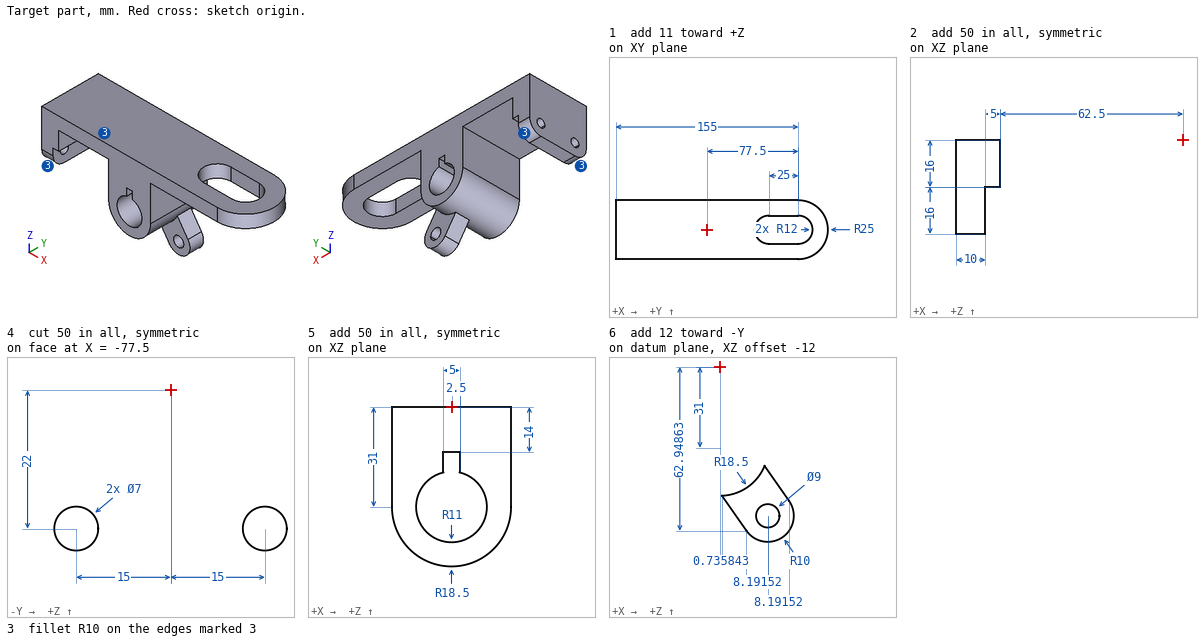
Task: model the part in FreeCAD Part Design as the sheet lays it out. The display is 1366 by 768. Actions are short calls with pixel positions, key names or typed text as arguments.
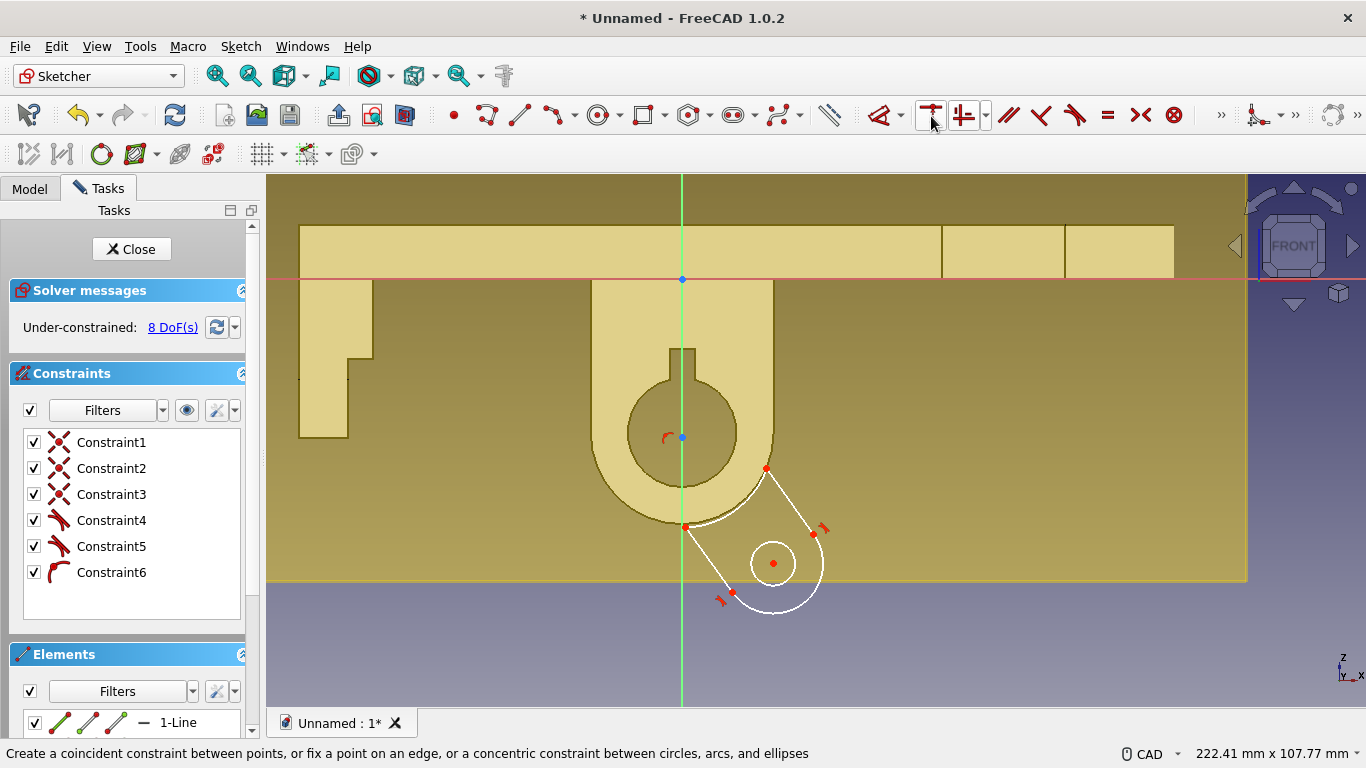
click(878, 116)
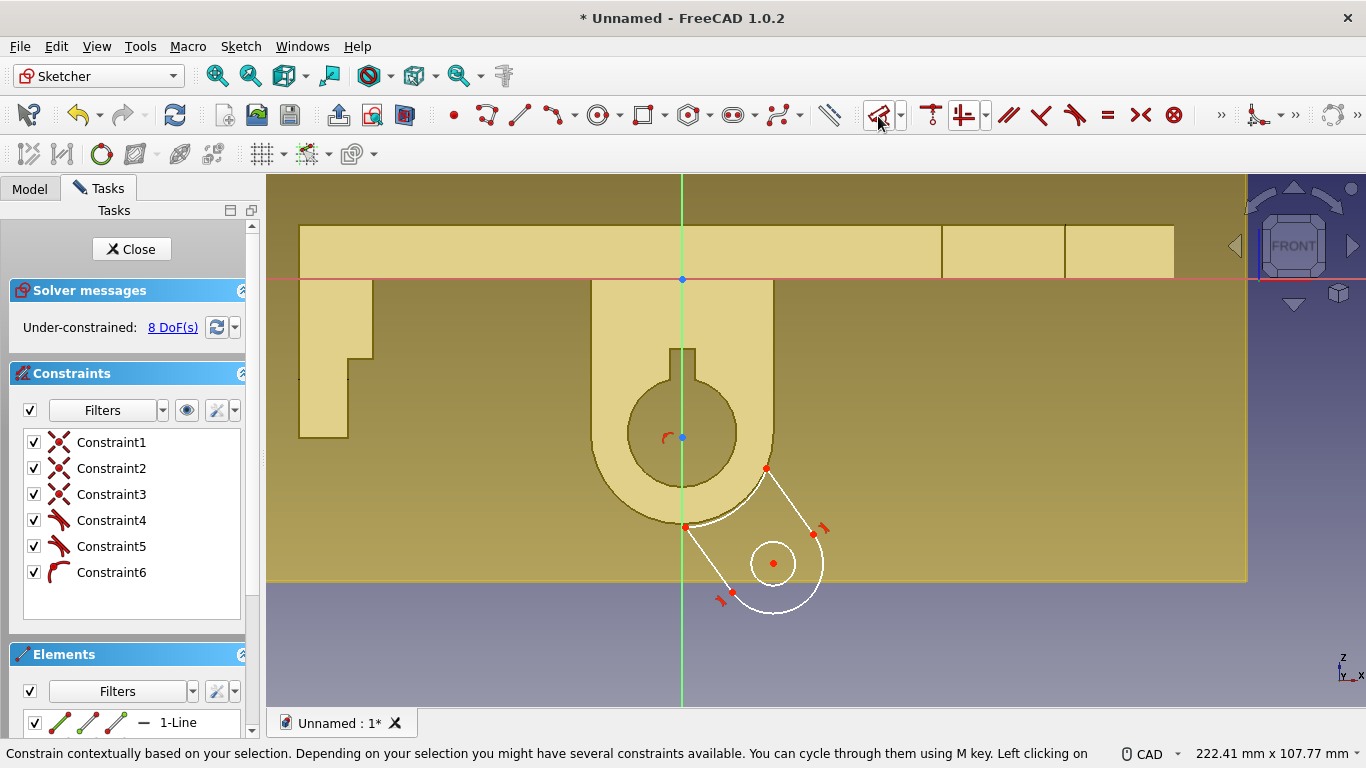
click(773, 614)
click(773, 646)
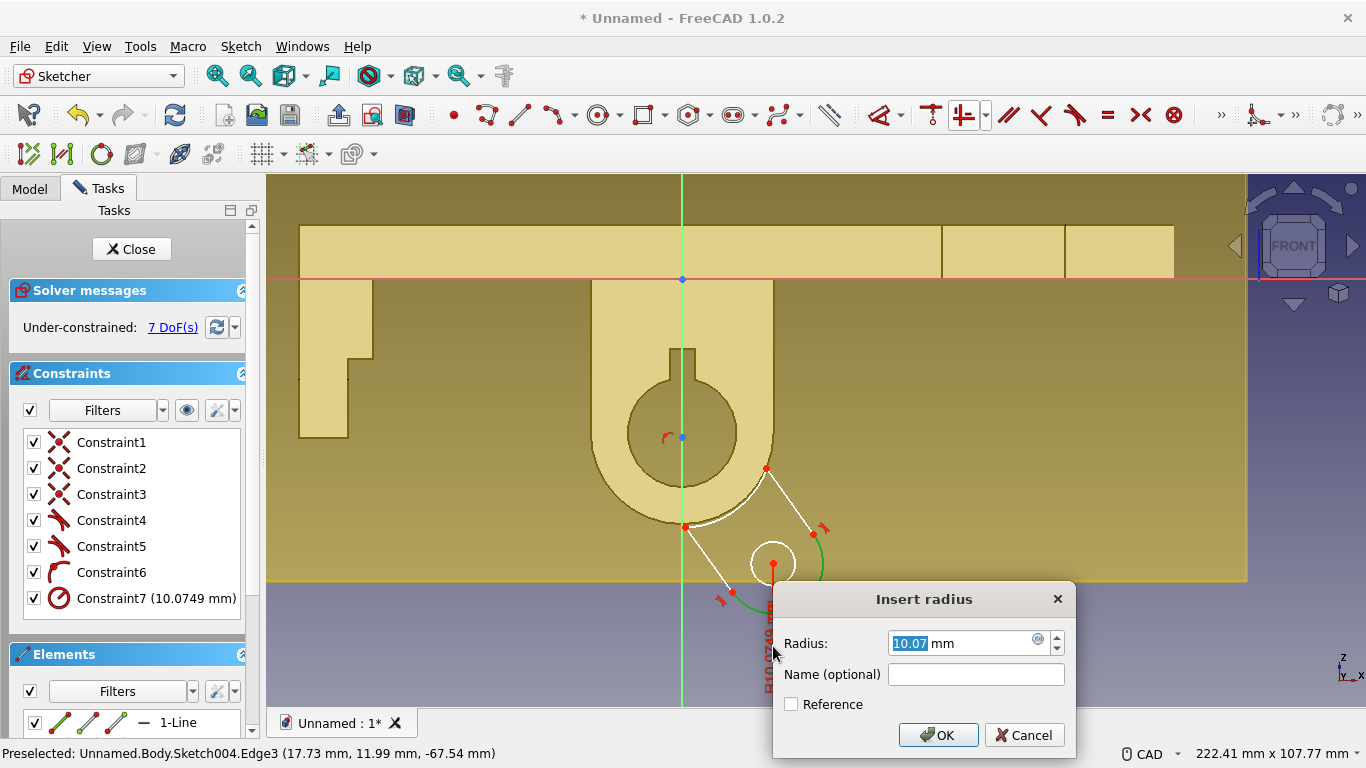
text(10)
key(Return)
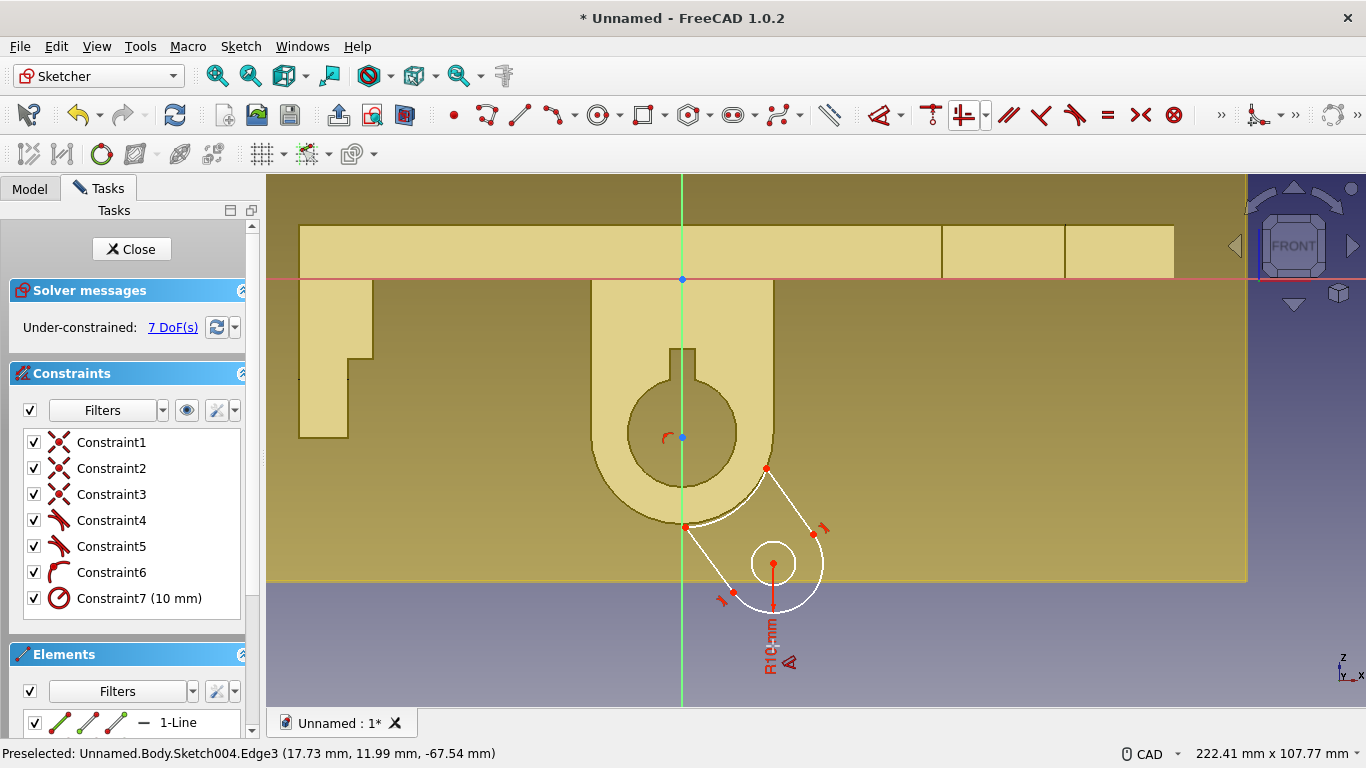
click(717, 521)
click(729, 551)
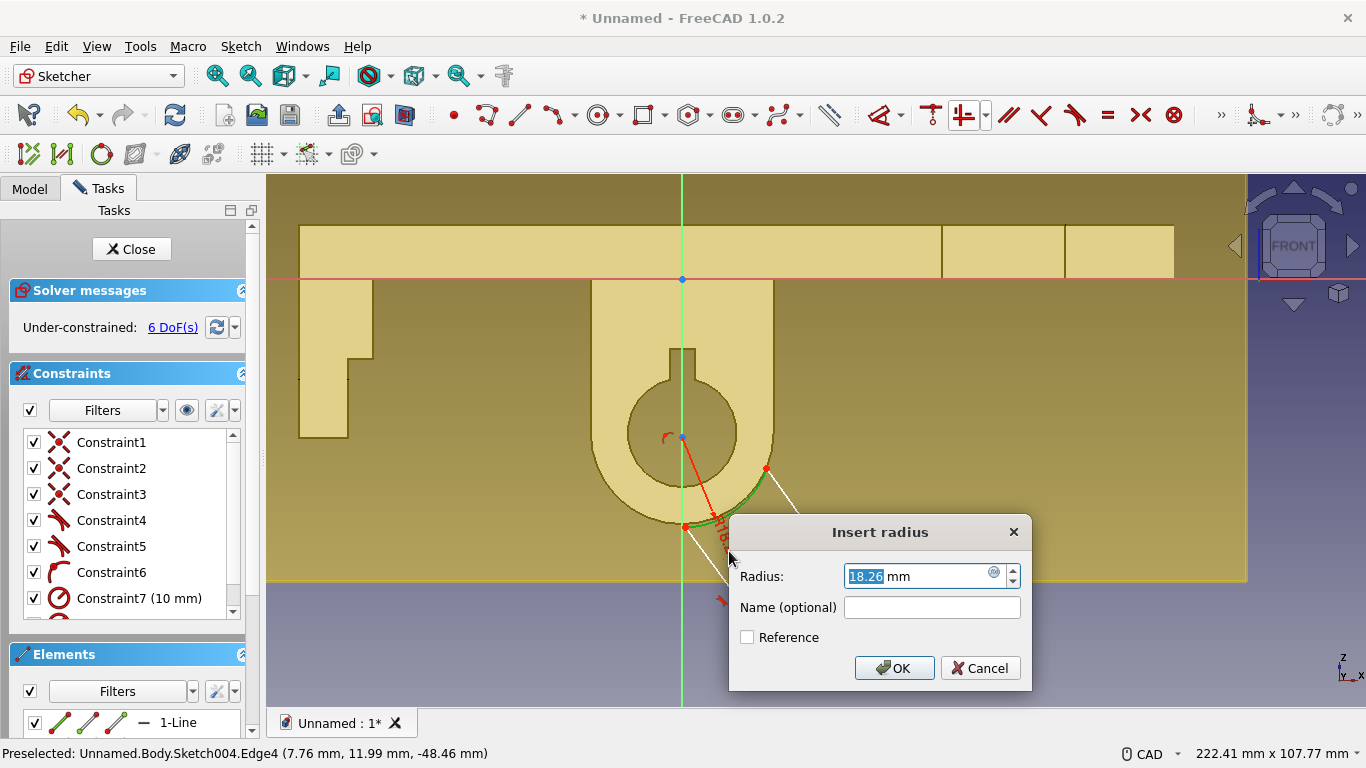
text(18.5)
key(Return)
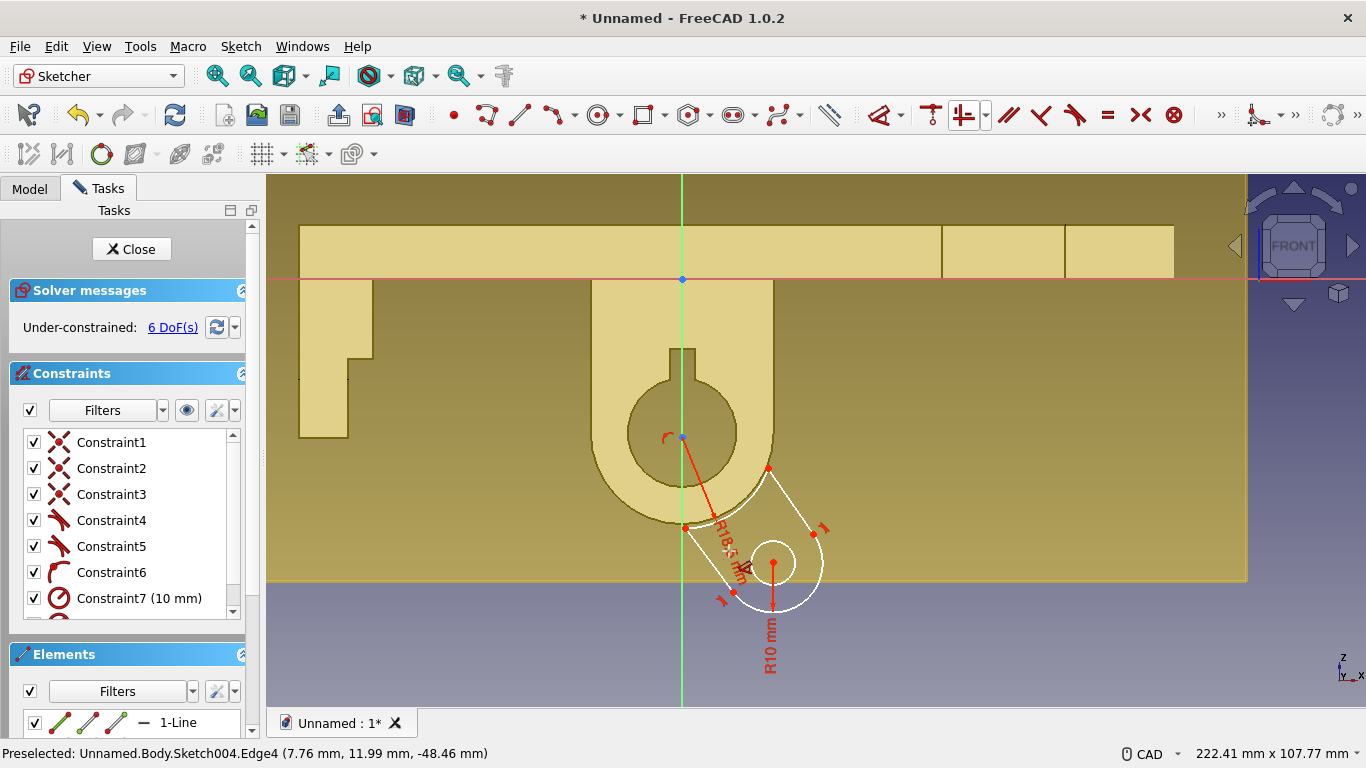
click(789, 547)
click(761, 510)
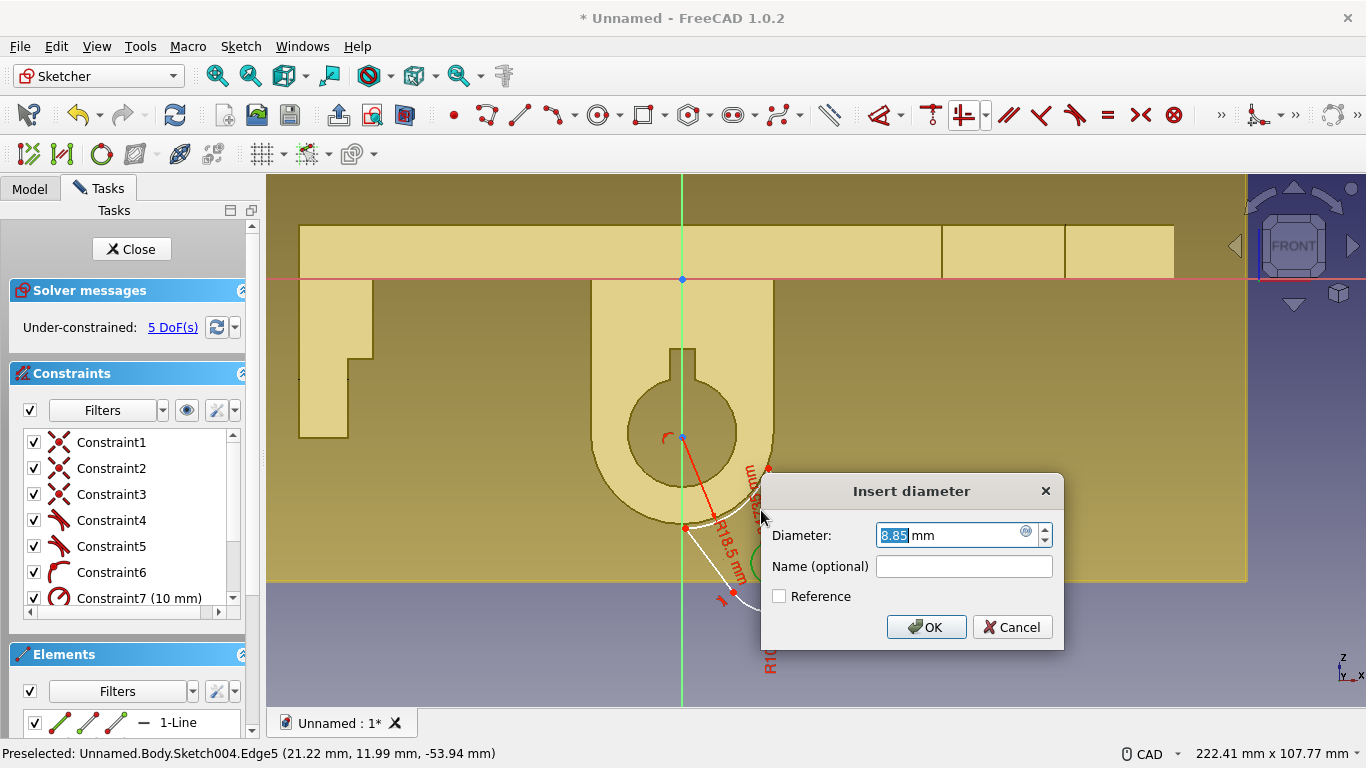
text(9)
key(Return)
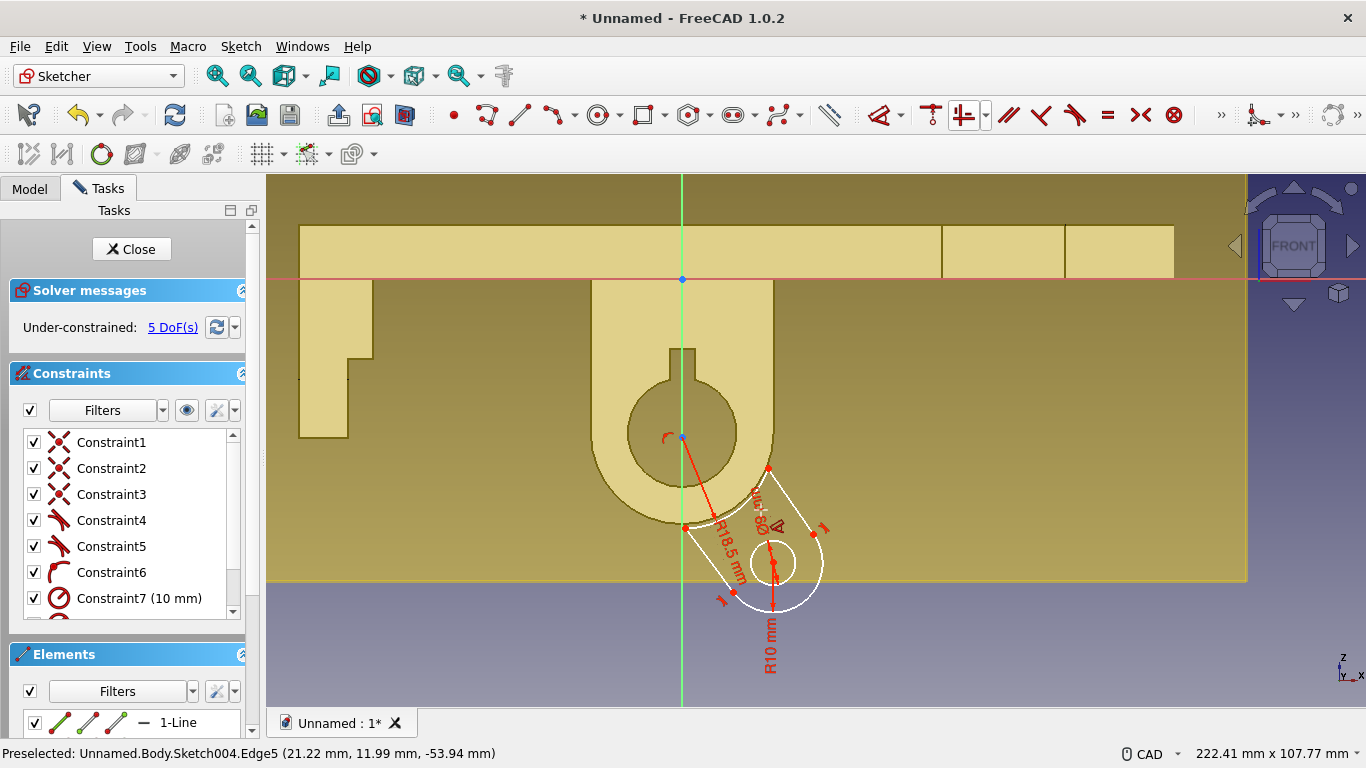
click(682, 437)
click(648, 358)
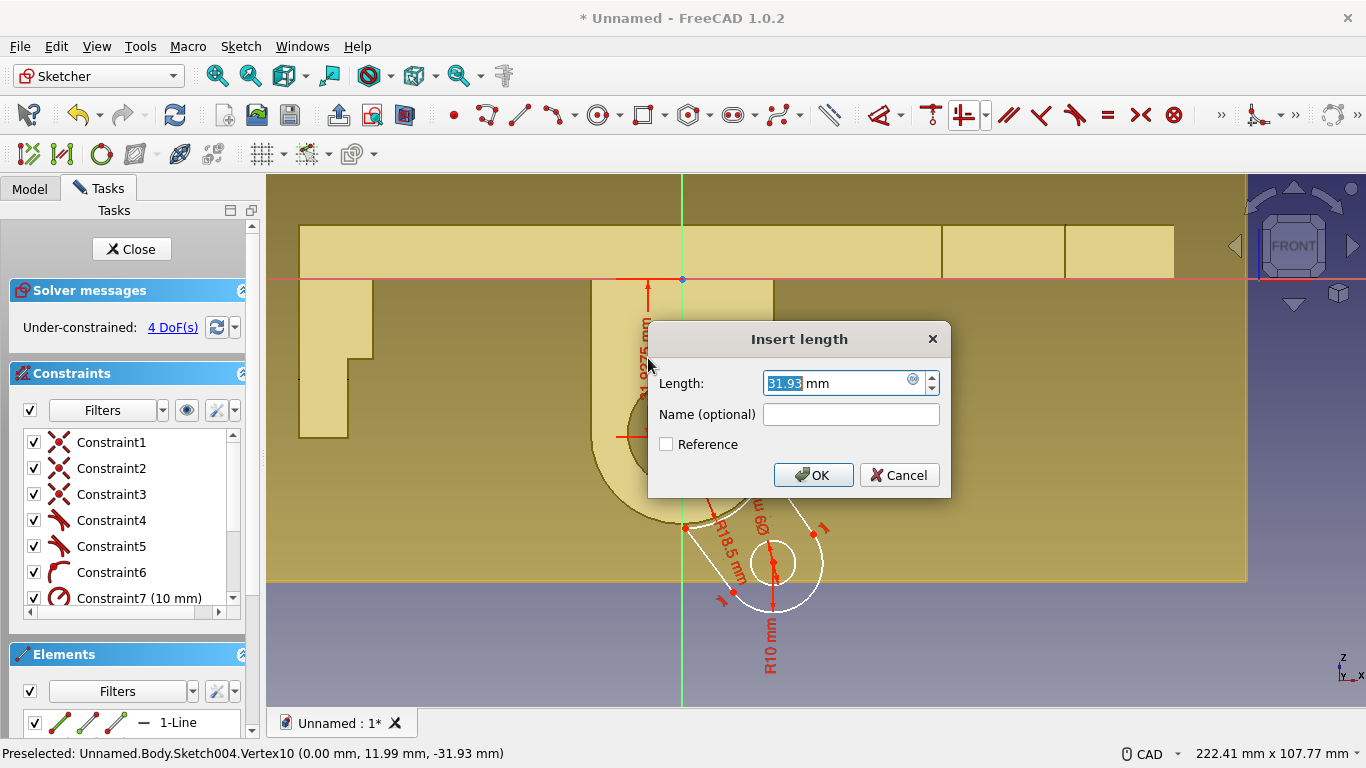
text(31)
key(Return)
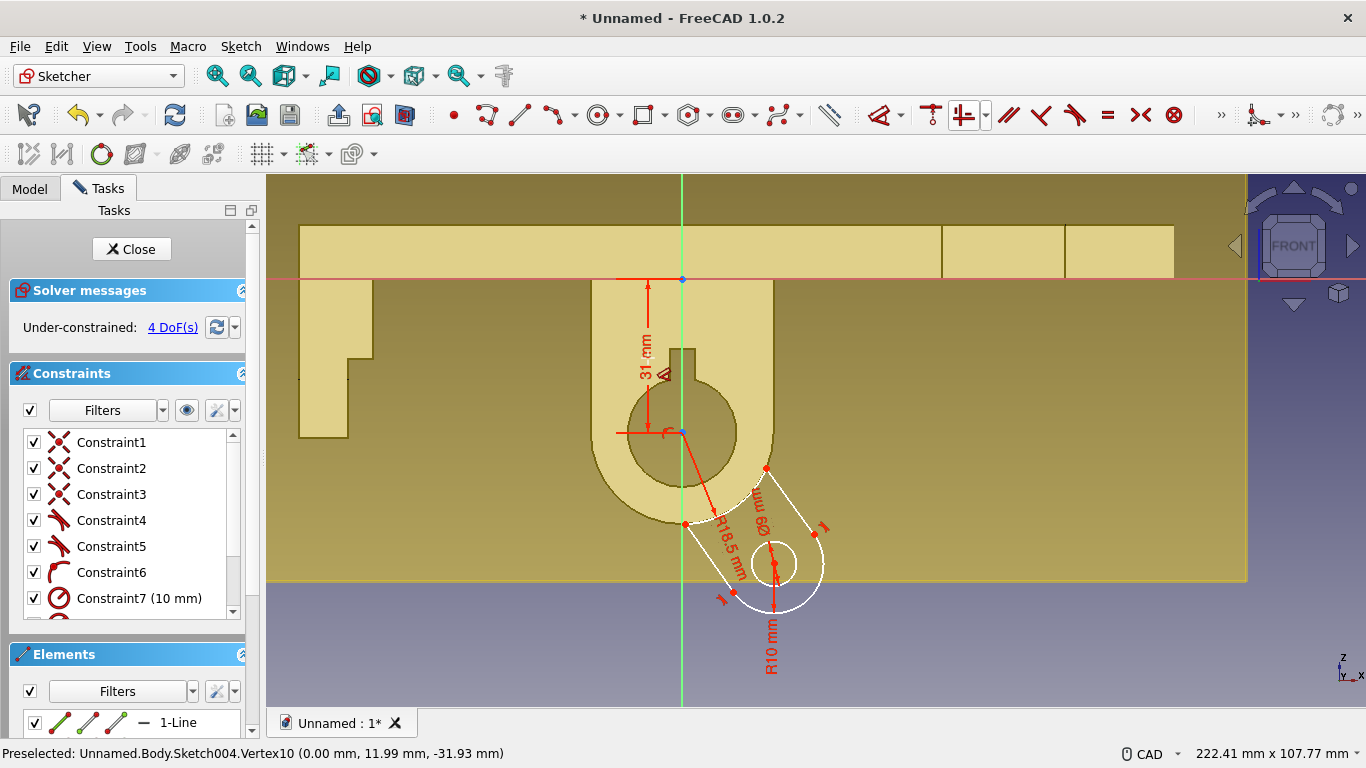
click(814, 535)